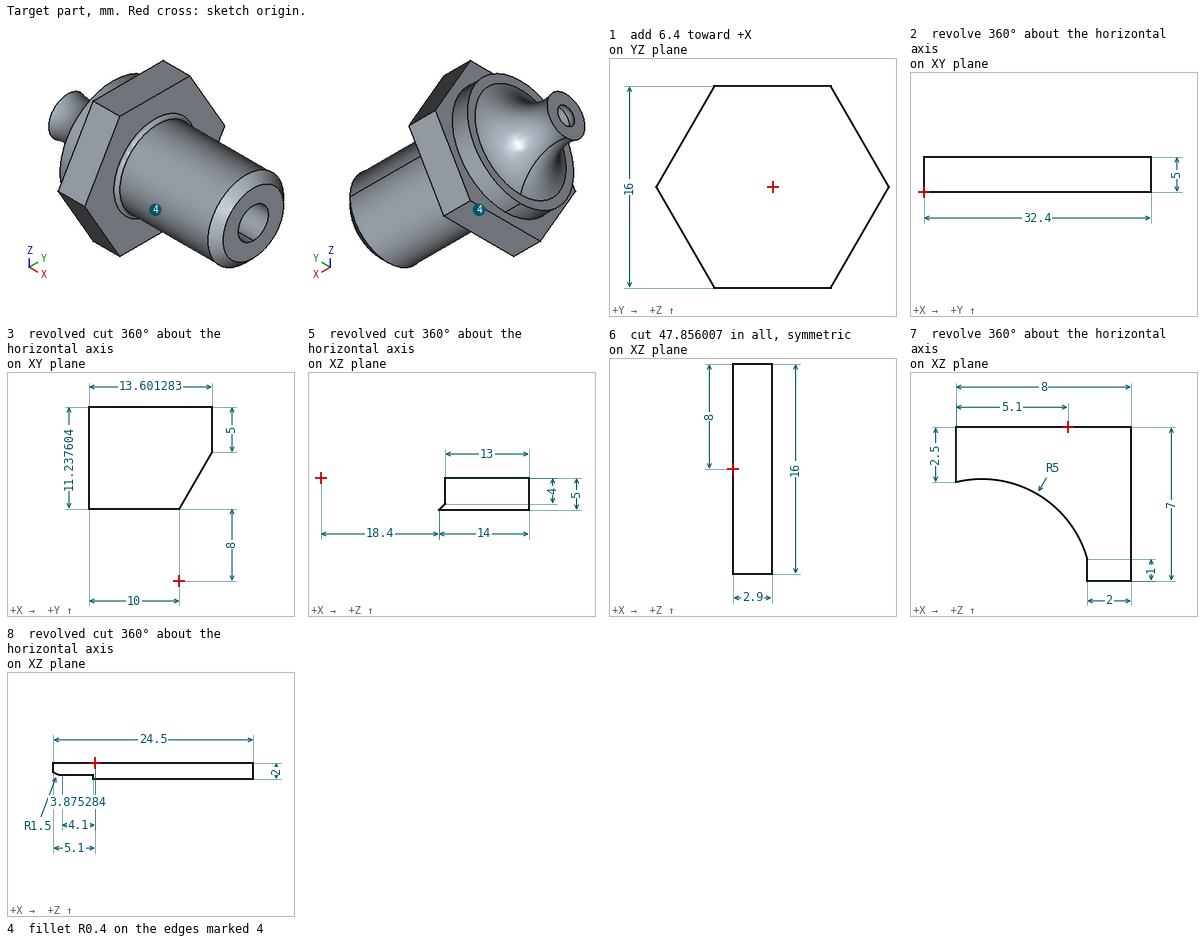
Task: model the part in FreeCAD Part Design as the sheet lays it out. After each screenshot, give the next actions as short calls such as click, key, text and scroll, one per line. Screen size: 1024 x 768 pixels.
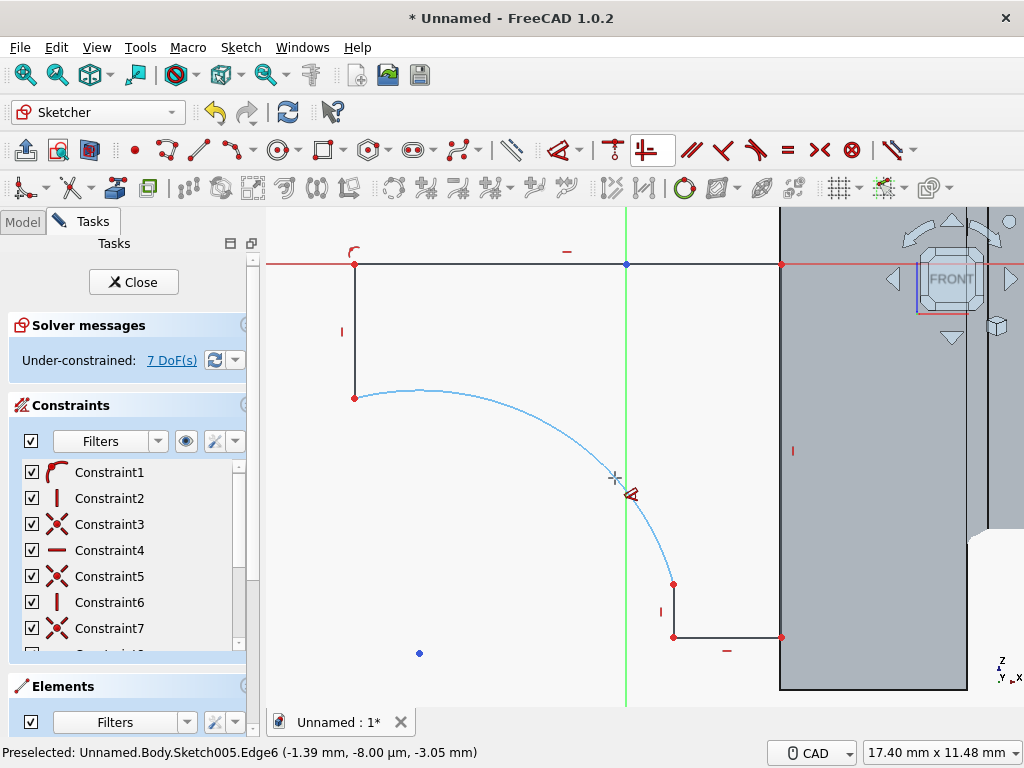
click(615, 477)
click(737, 642)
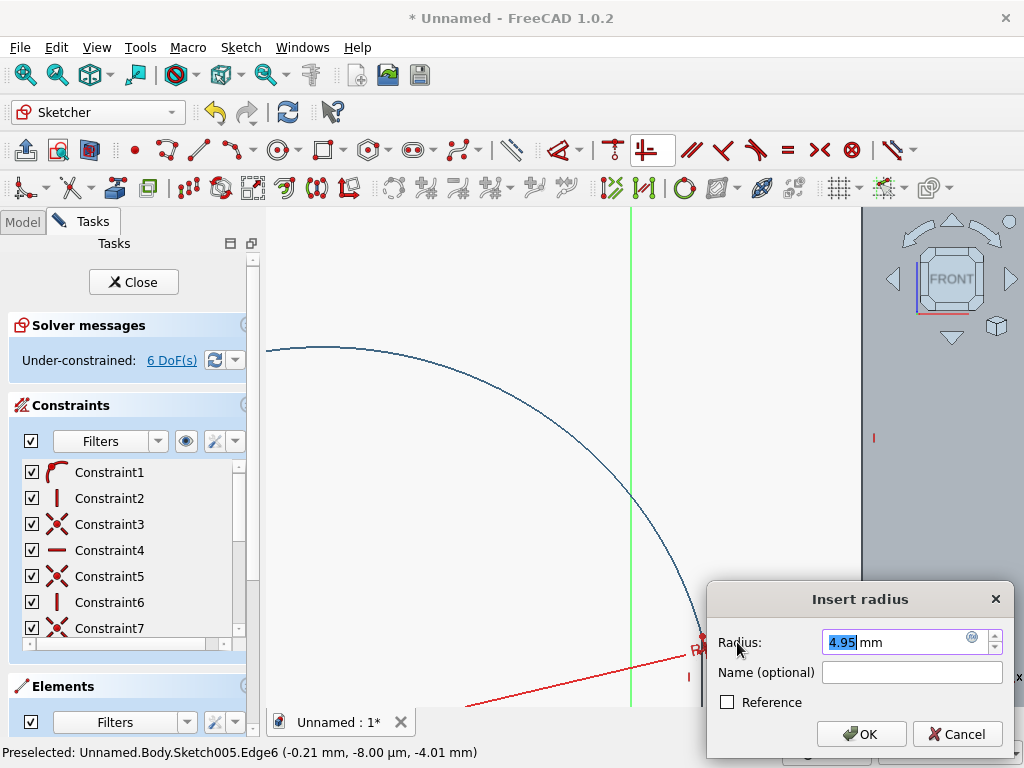
text(5)
key(Return)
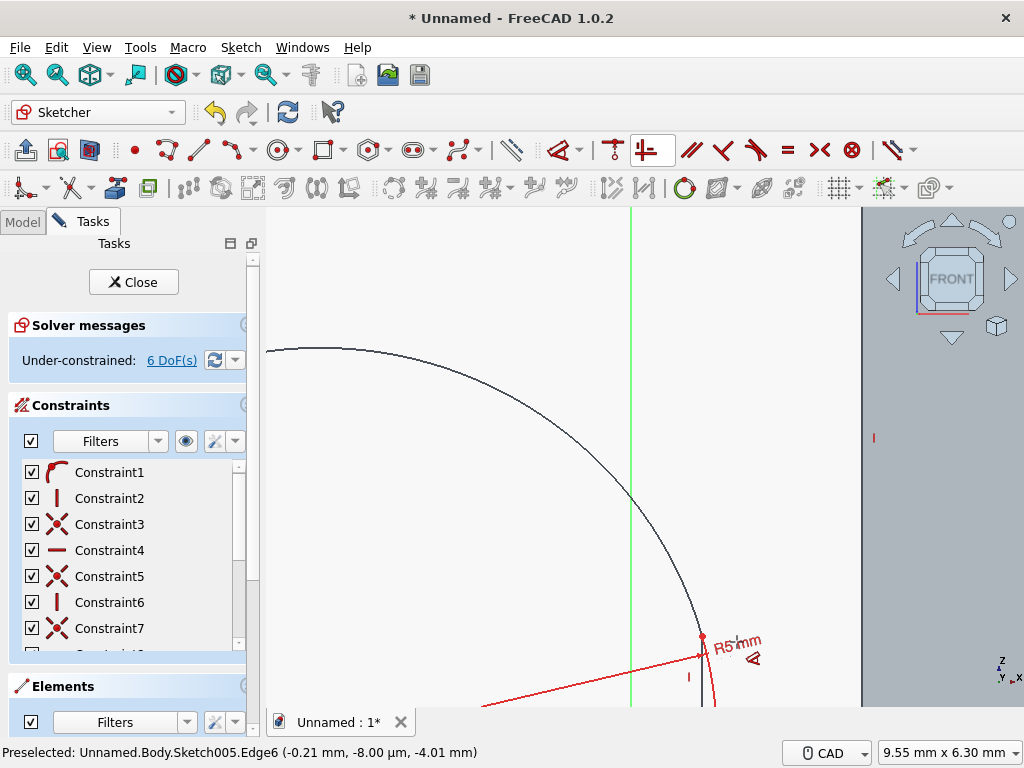
scroll(616, 482, down, 3)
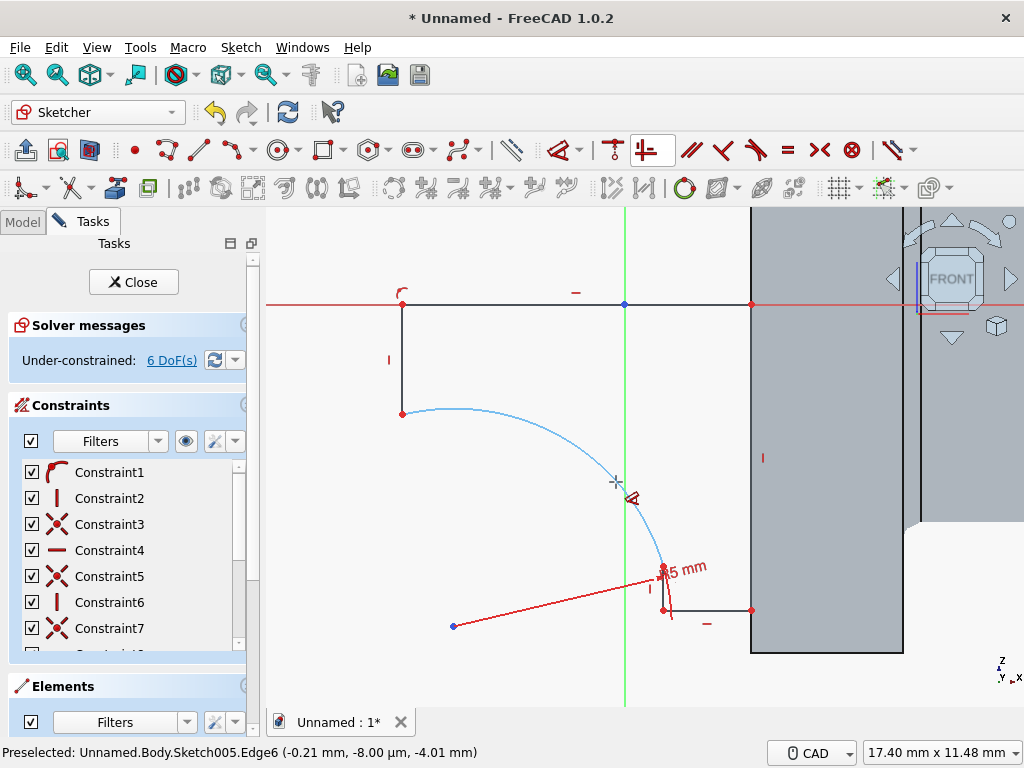
click(507, 305)
click(577, 271)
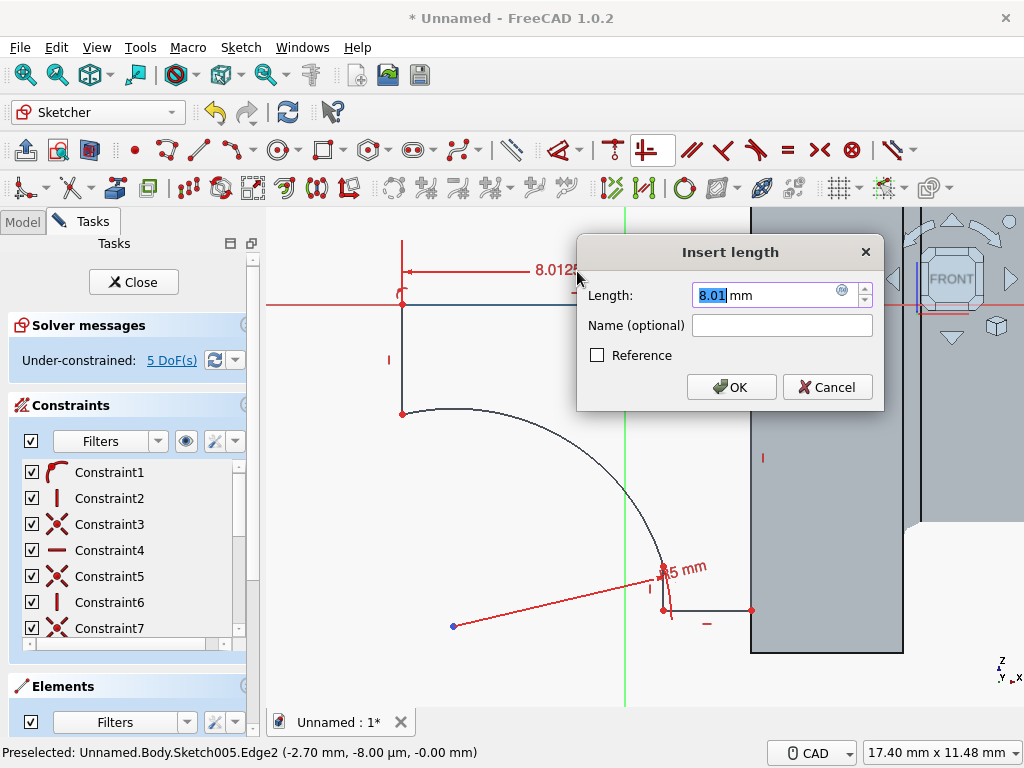
text(8)
key(Return)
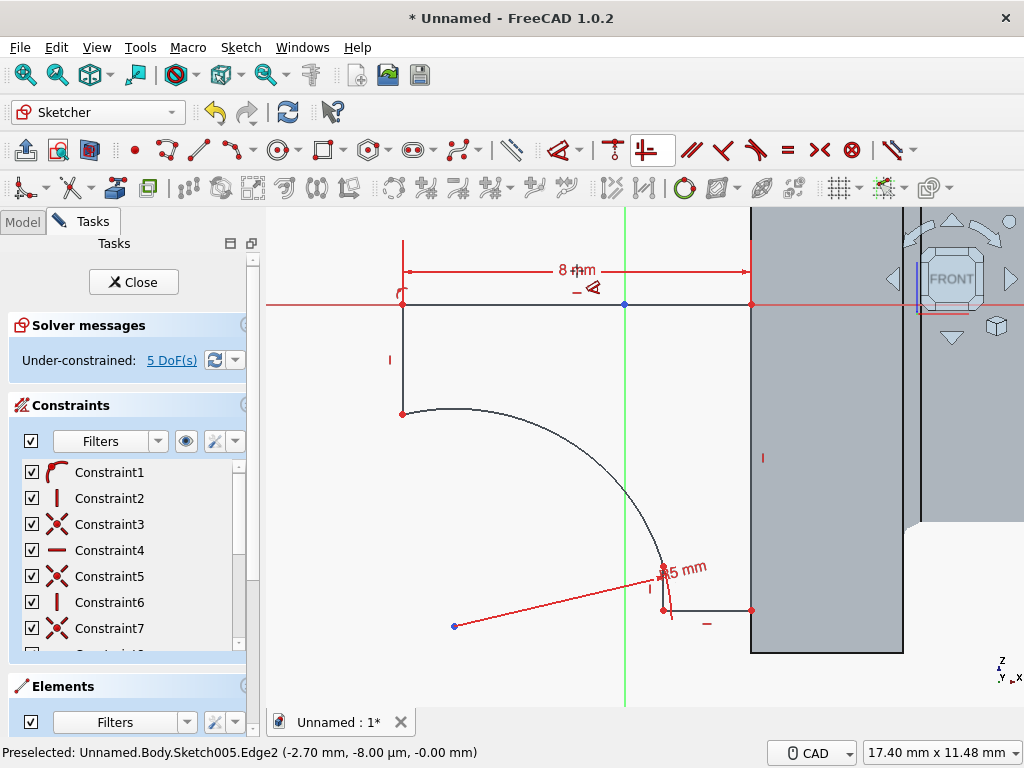
click(751, 397)
click(785, 458)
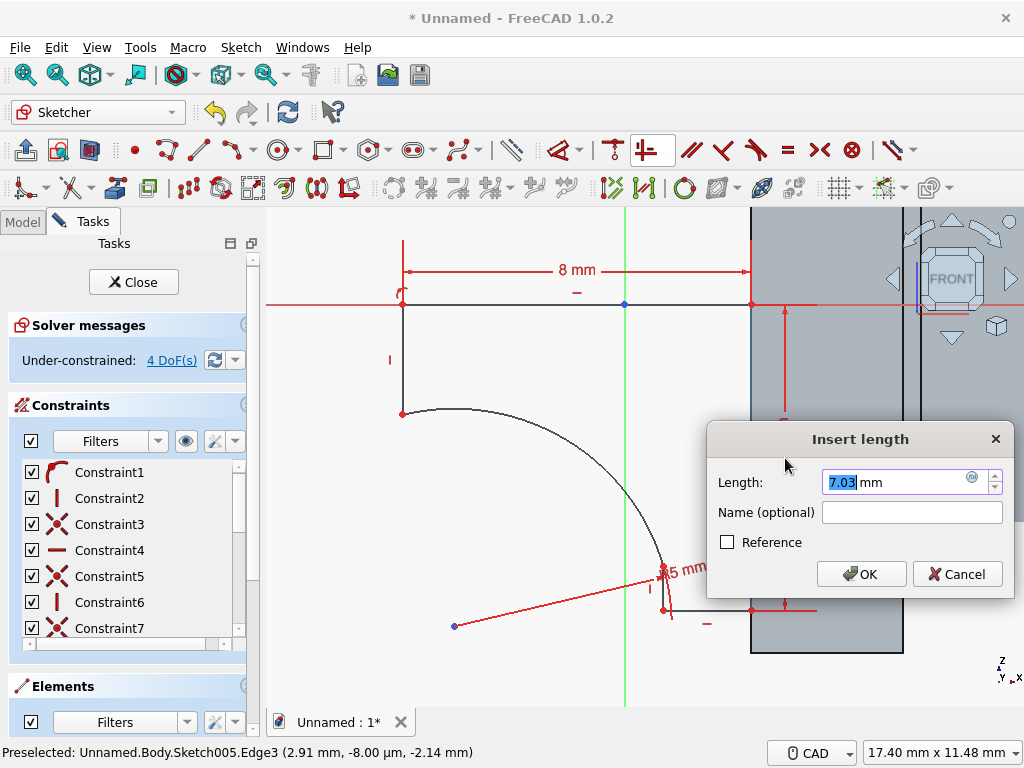
text(7)
key(Return)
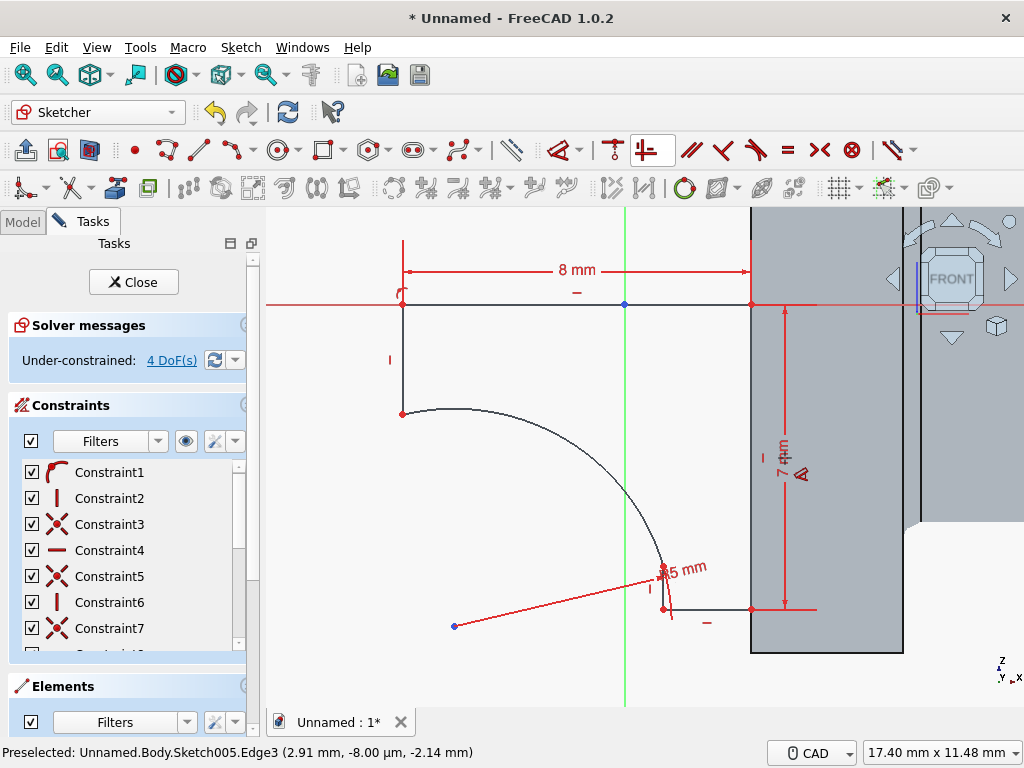
click(725, 610)
click(707, 644)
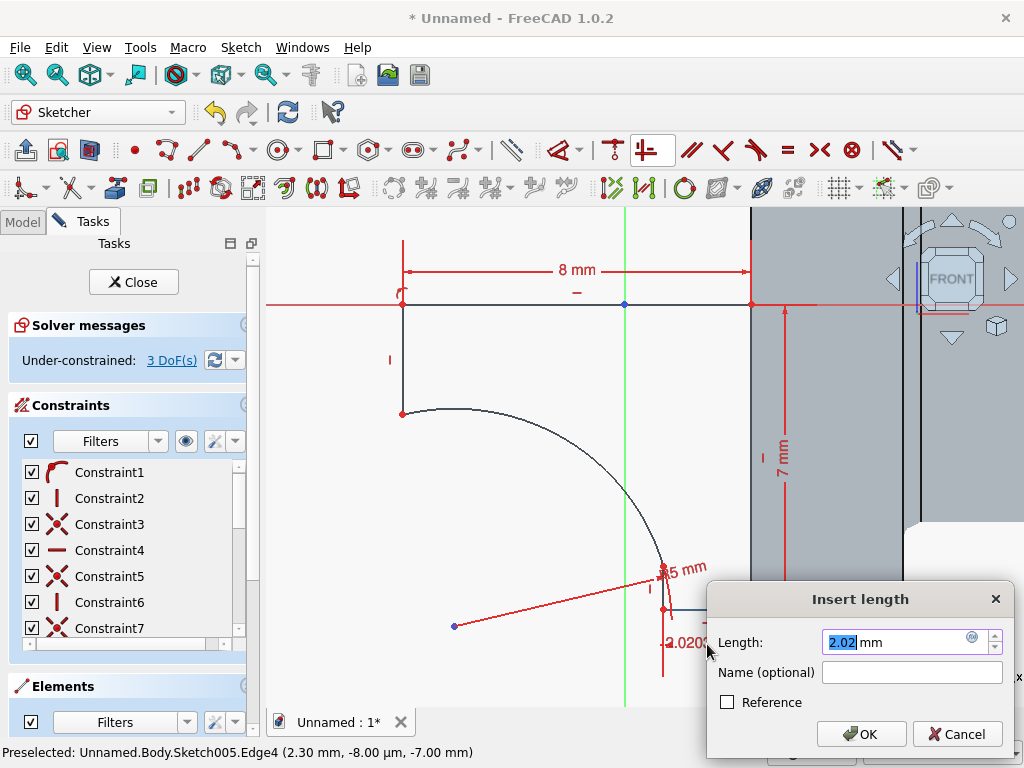
text(2)
key(Return)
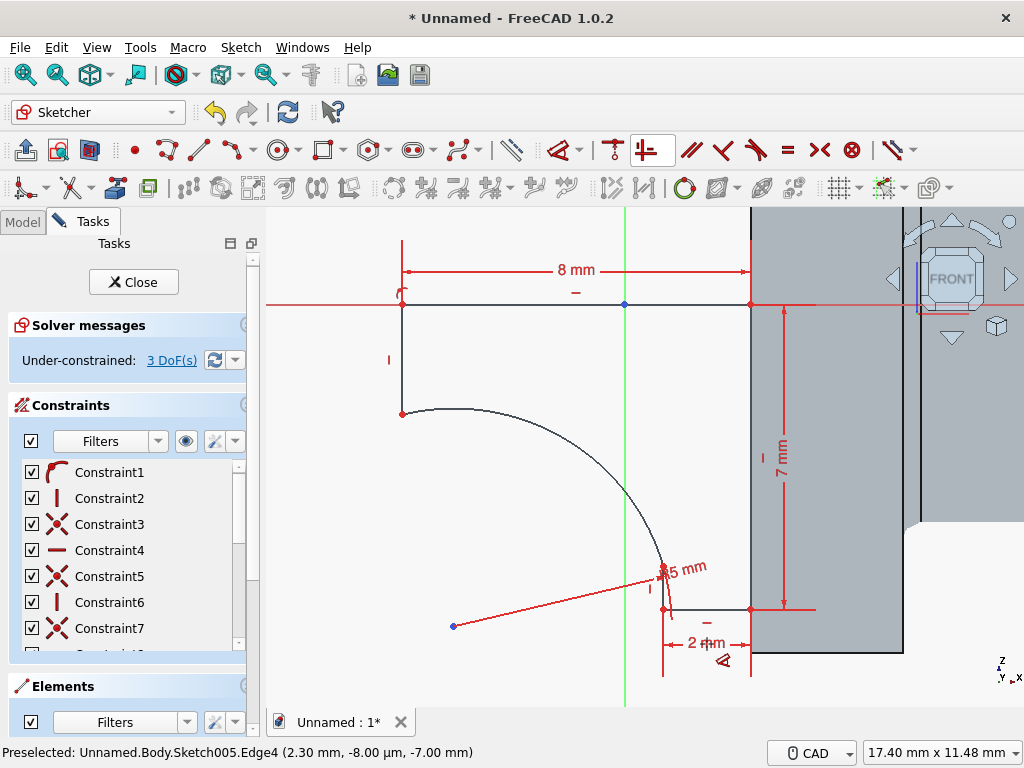
click(663, 597)
click(605, 588)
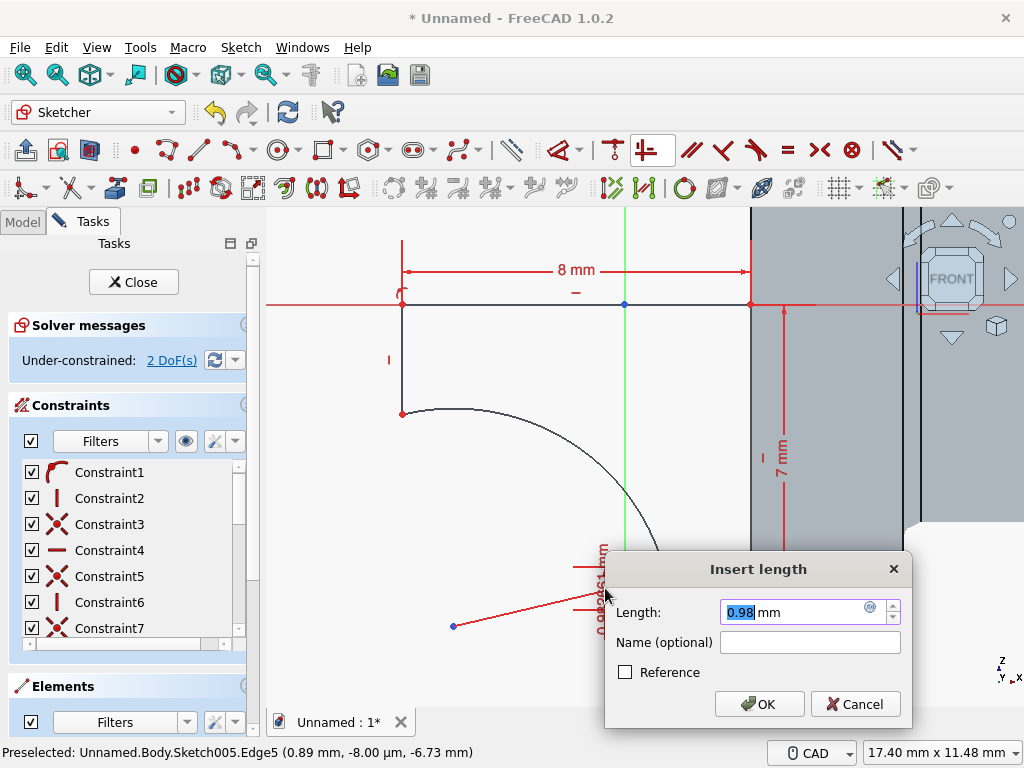
text(1)
key(Return)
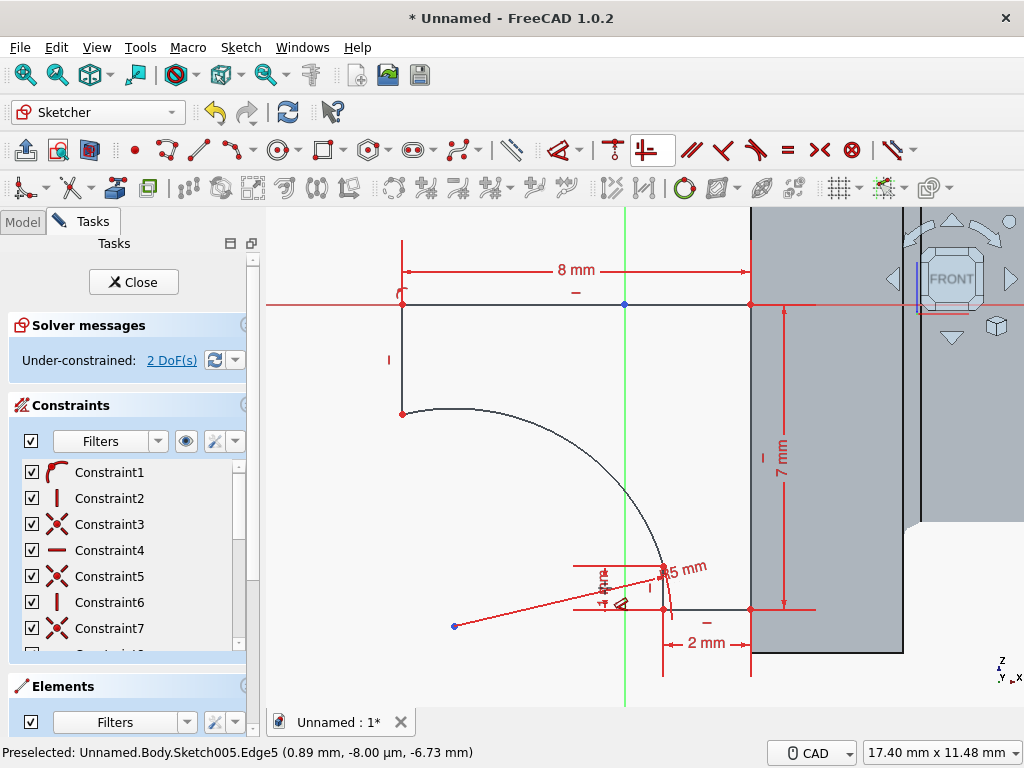
click(402, 382)
click(368, 360)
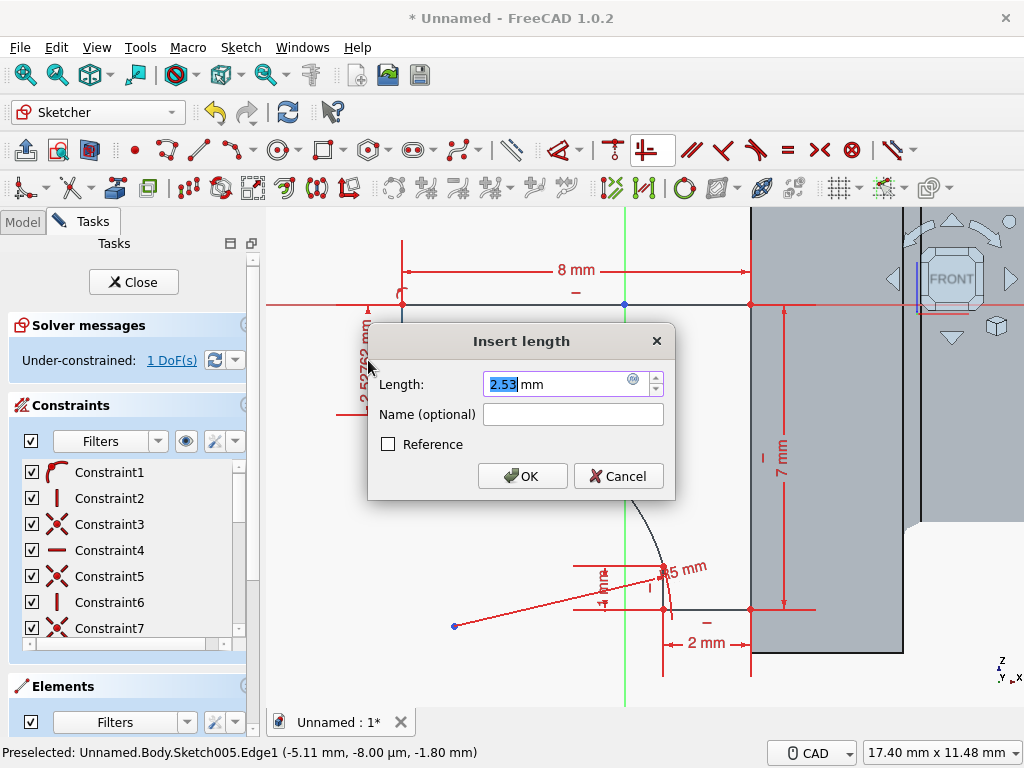
text(2.5)
key(Return)